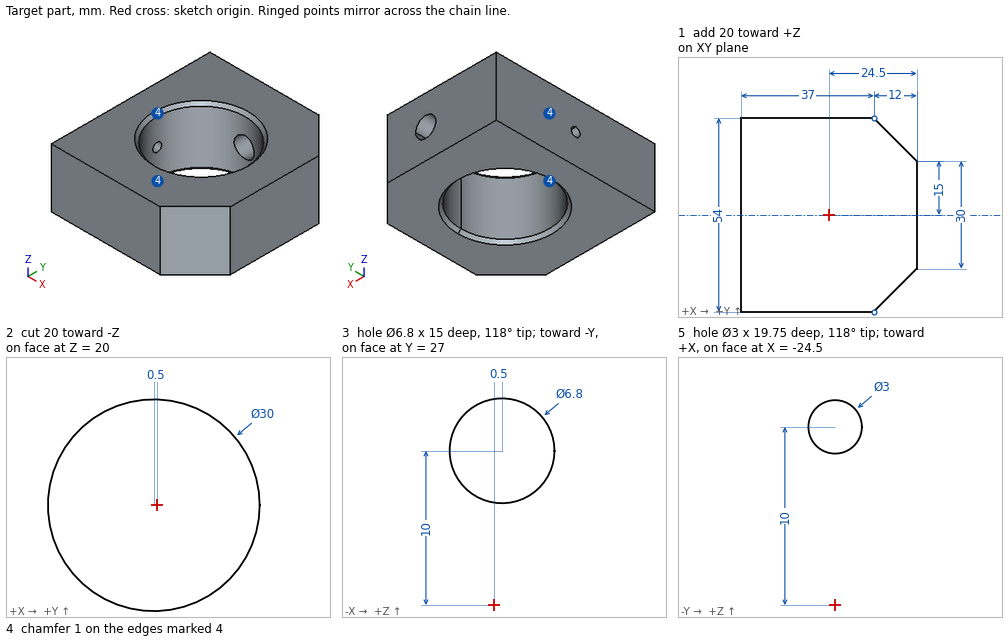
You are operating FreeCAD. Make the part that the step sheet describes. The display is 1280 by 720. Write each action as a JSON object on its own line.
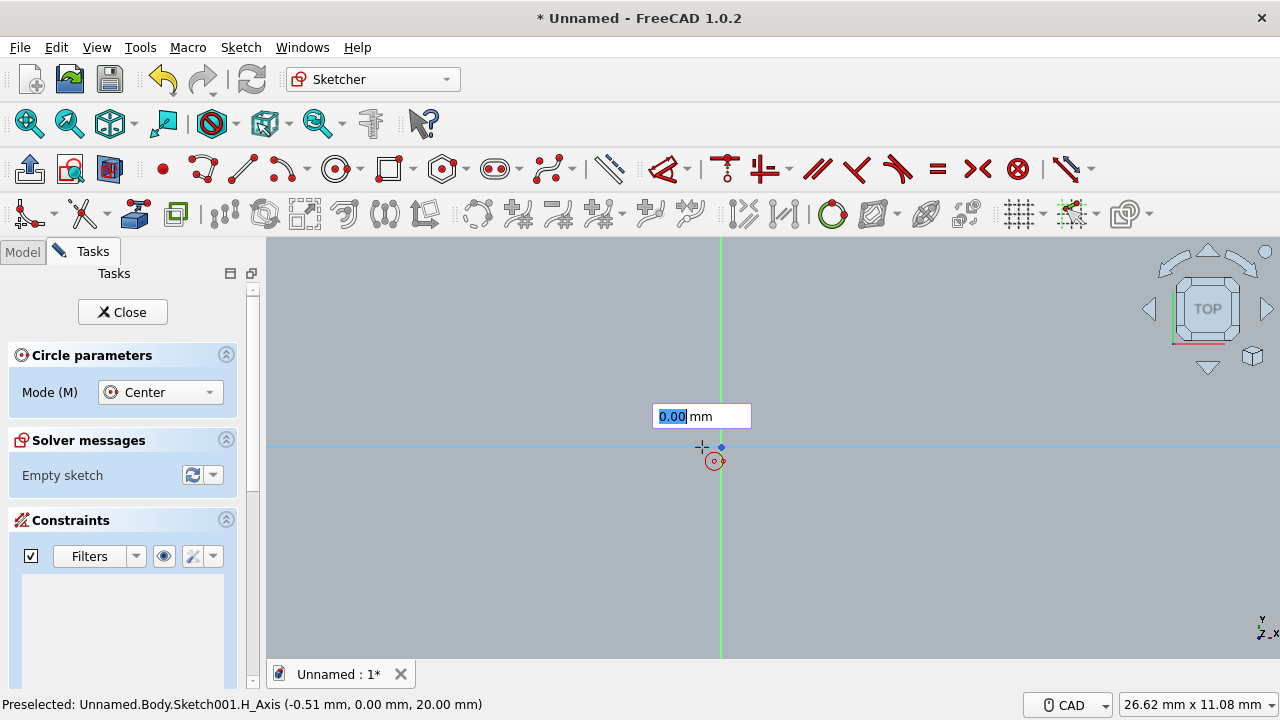
{"action": "scroll", "coordinate": [705, 448], "scroll_direction": "down", "scroll_amount": 7}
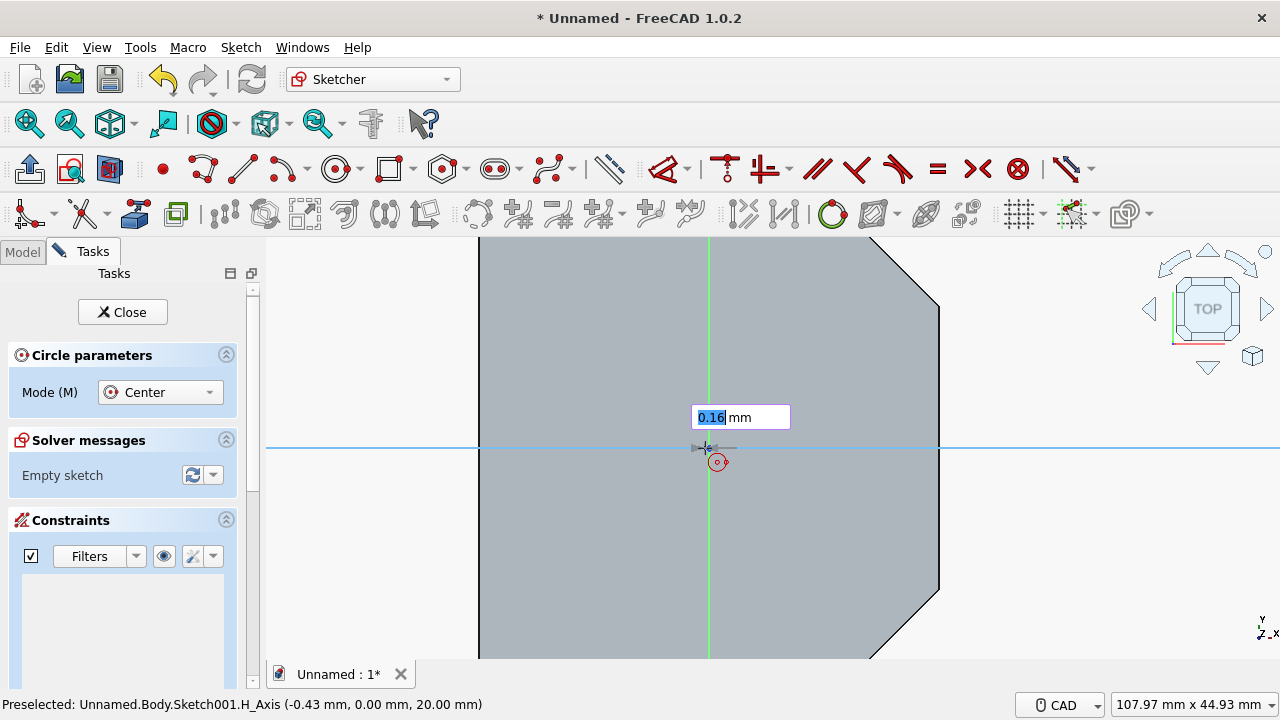
{"action": "left_click", "coordinate": [804, 349]}
{"action": "key", "text": "Escape"}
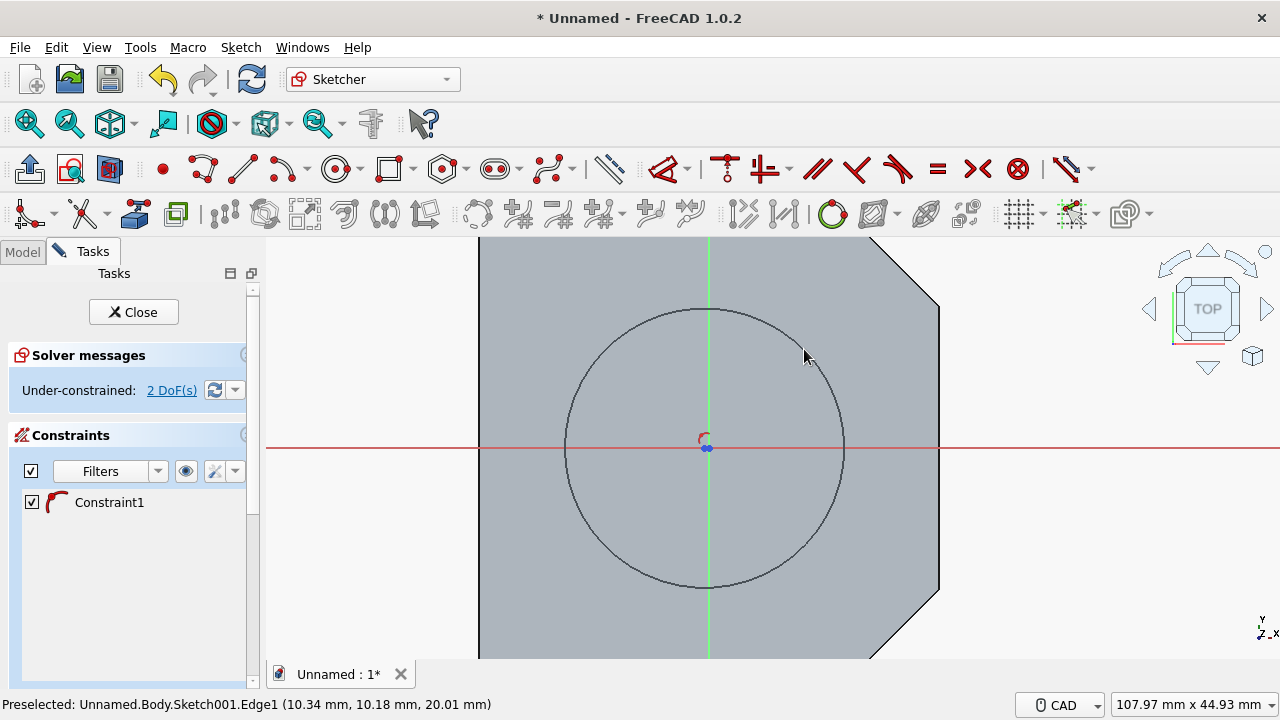
{"action": "key", "text": "d"}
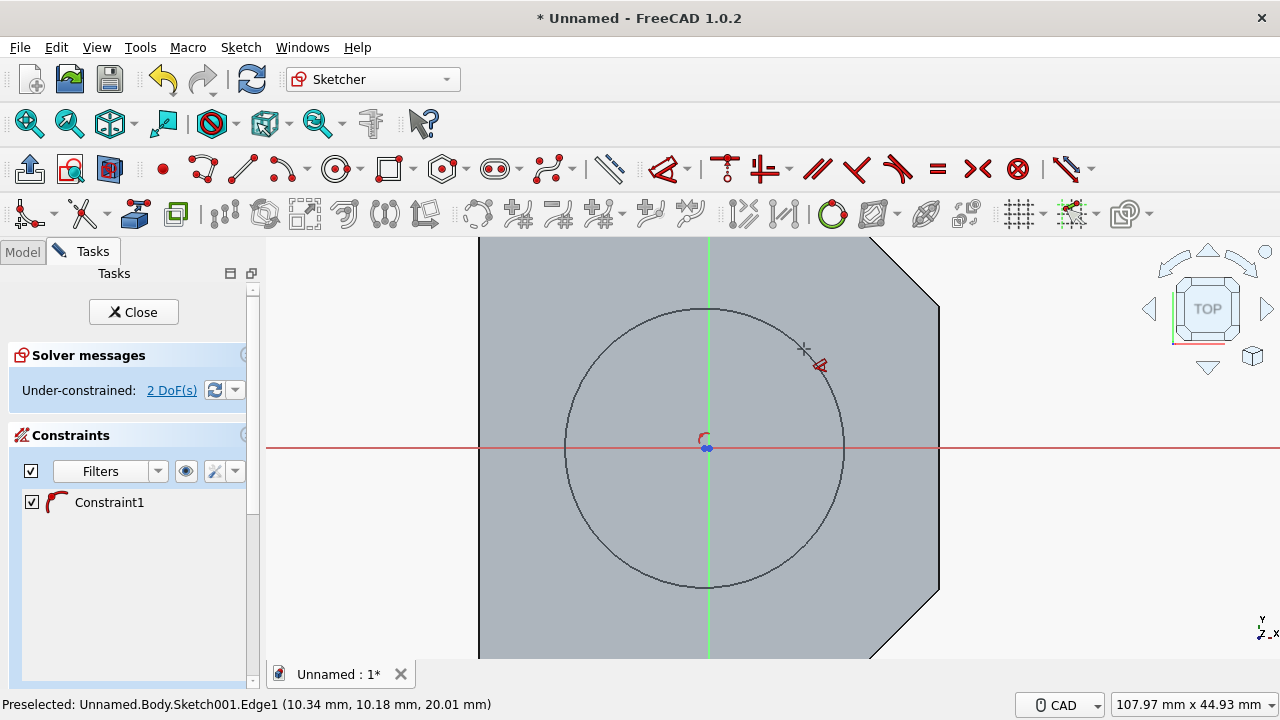
{"action": "left_click", "coordinate": [803, 349]}
{"action": "left_click", "coordinate": [826, 326]}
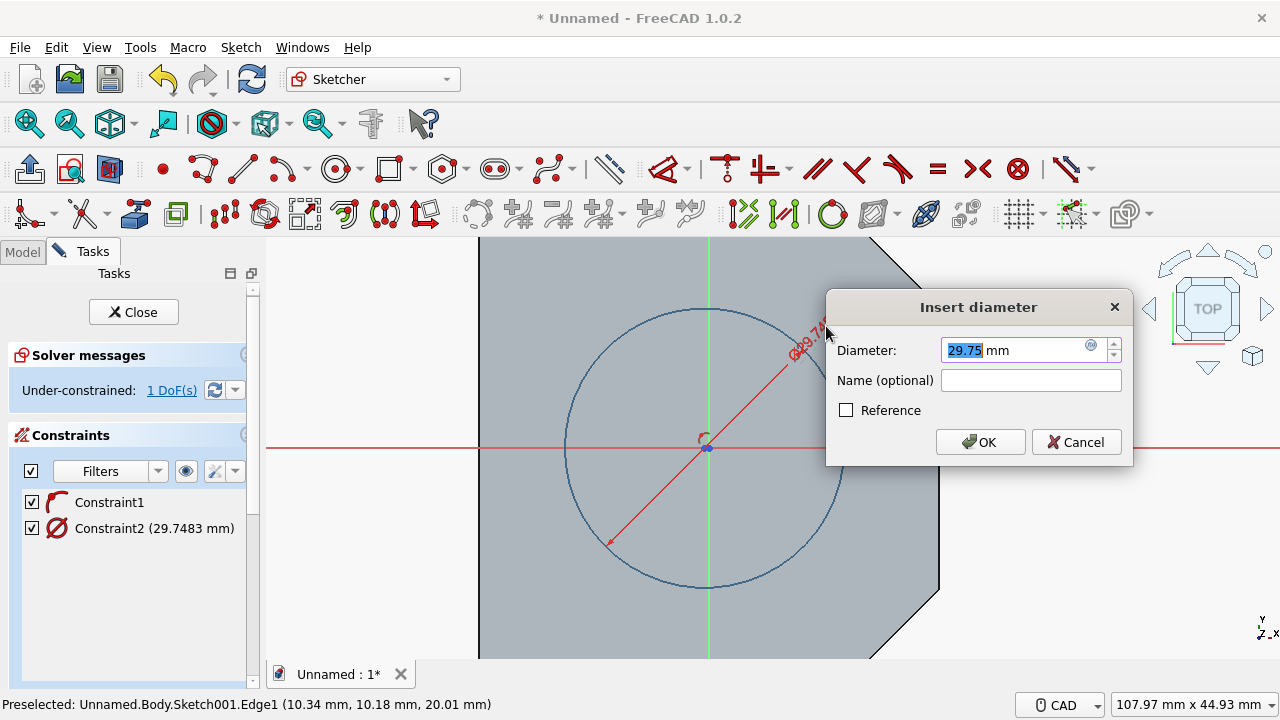
{"action": "type", "text": "30"}
{"action": "key", "text": "Return"}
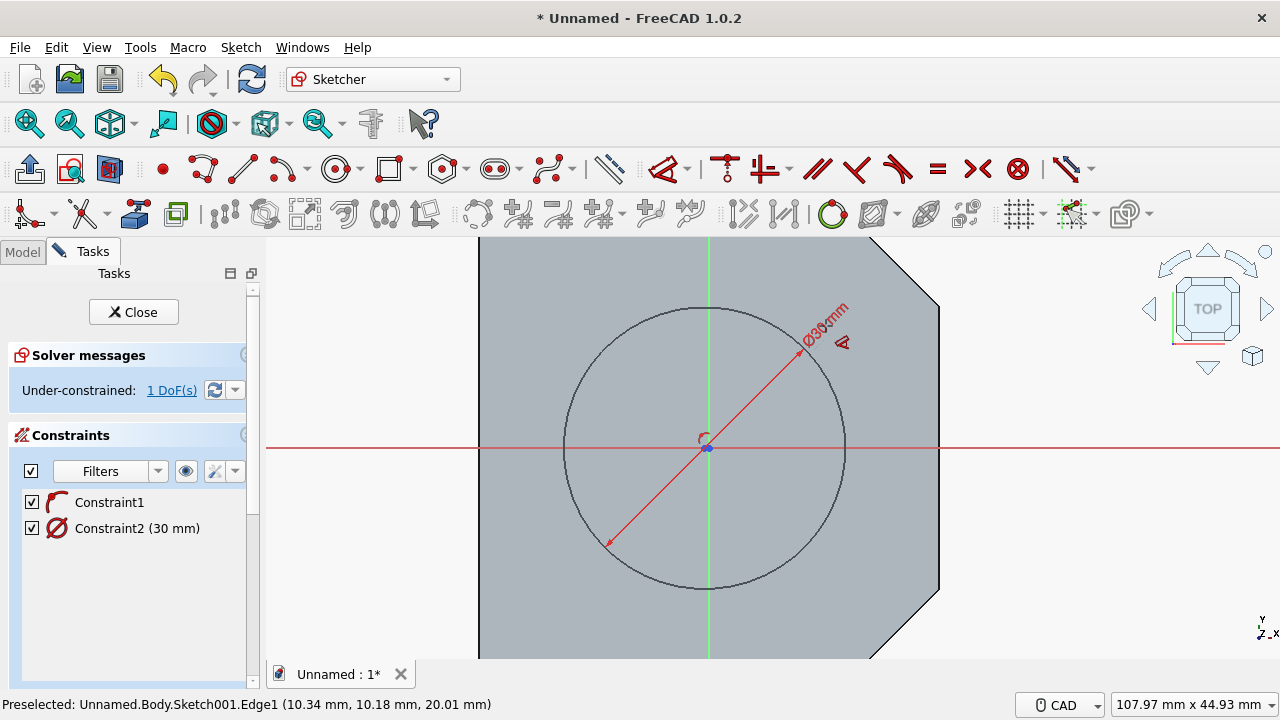
{"action": "scroll", "coordinate": [705, 448], "scroll_direction": "up", "scroll_amount": 11}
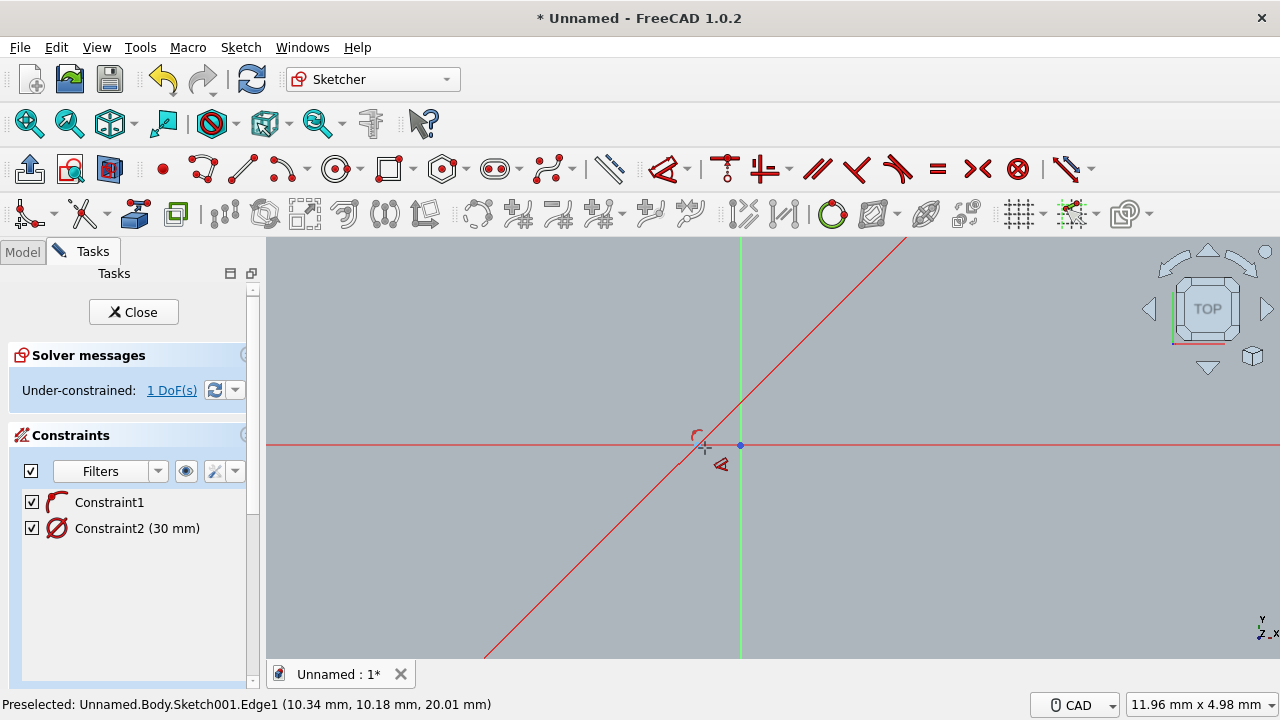
{"action": "left_click", "coordinate": [698, 445]}
{"action": "left_click", "coordinate": [719, 479]}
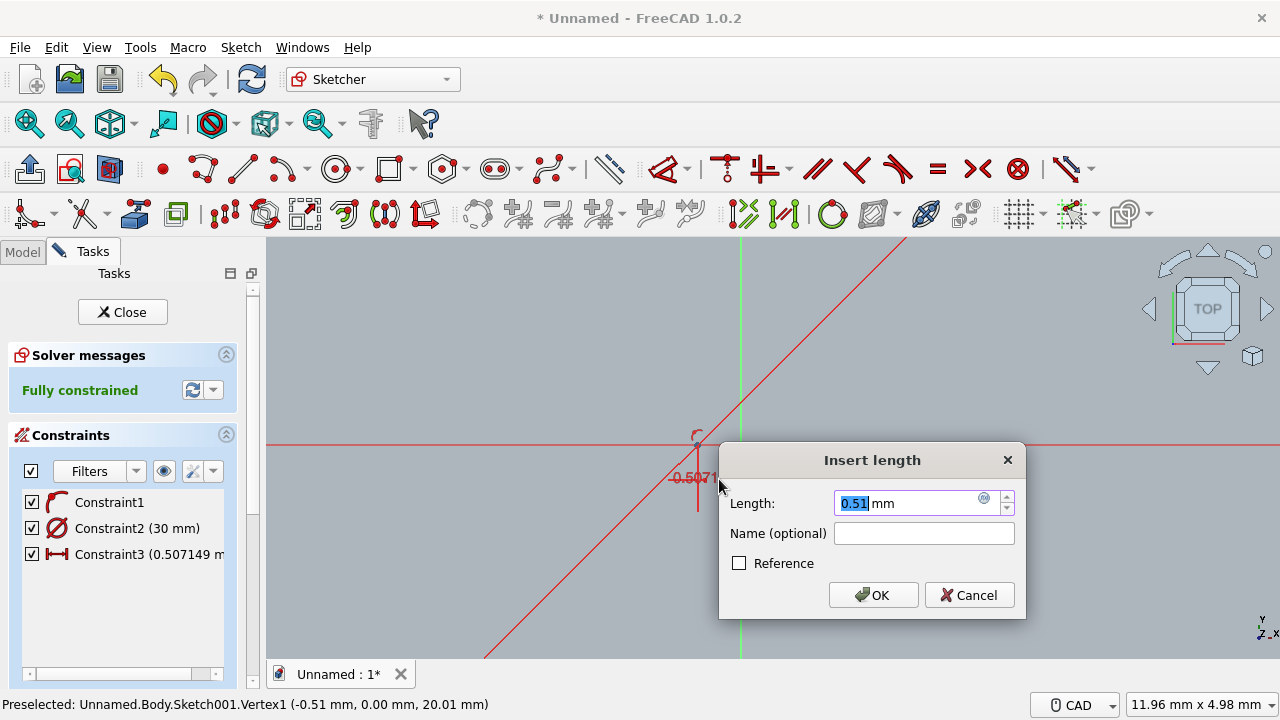
{"action": "type", "text": "0.5"}
{"action": "key", "text": "Return"}
{"action": "key", "text": "Escape"}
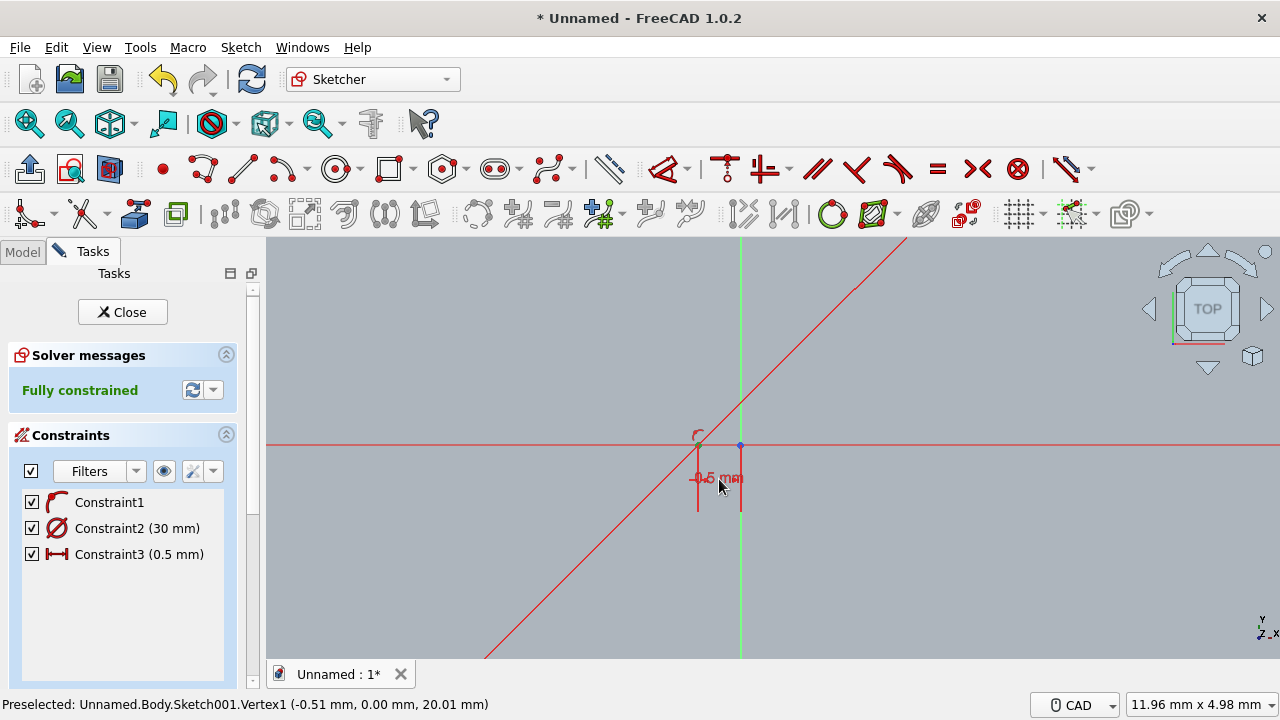
{"action": "left_click", "coordinate": [123, 312]}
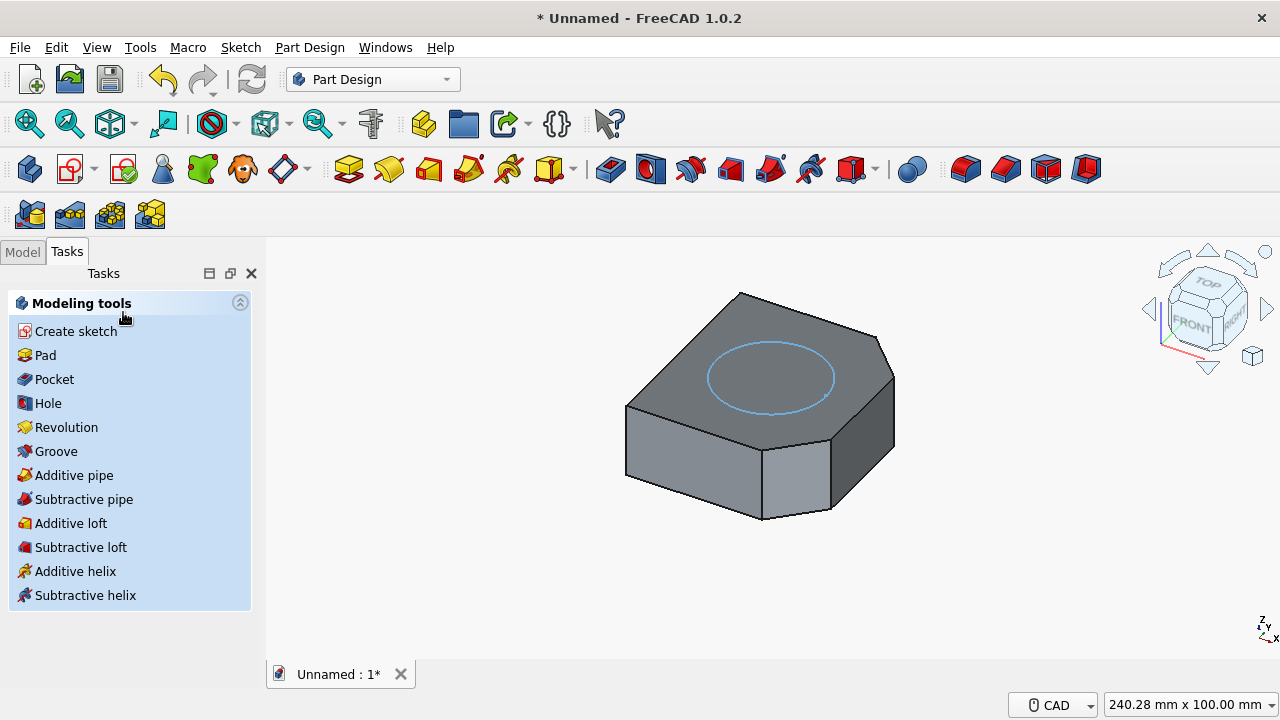
{"action": "left_click", "coordinate": [612, 170]}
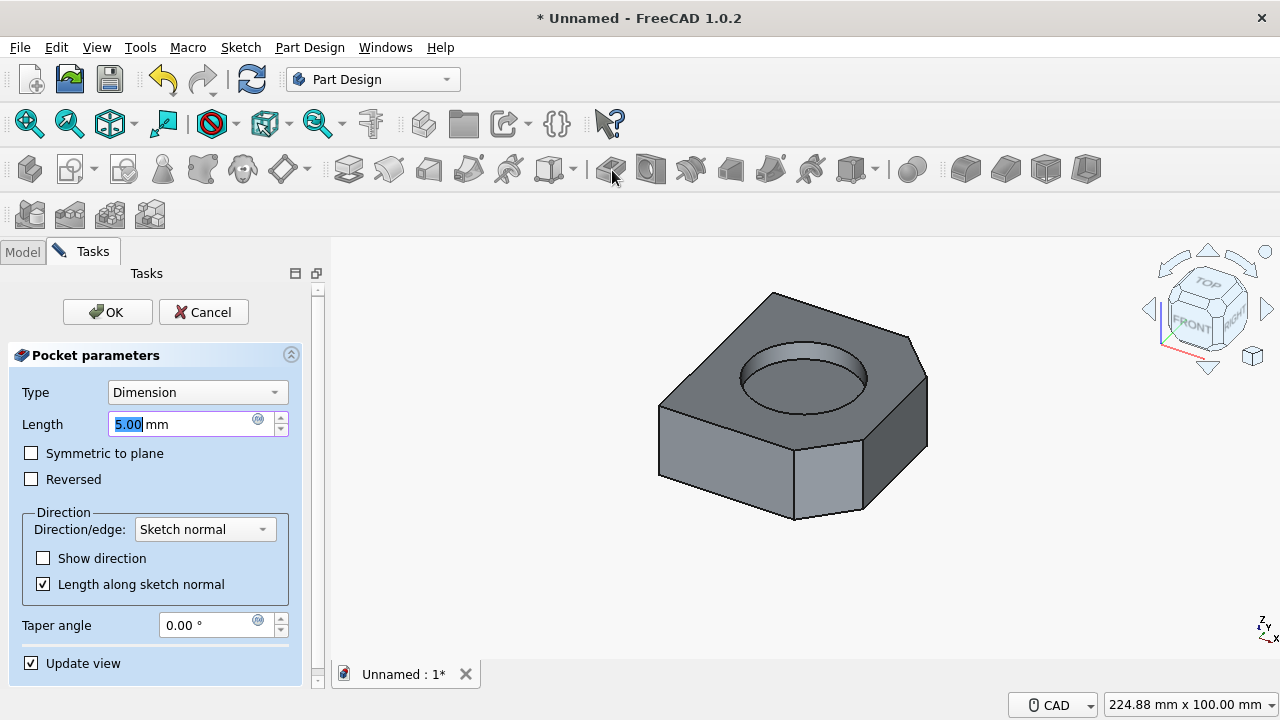
{"action": "type", "text": "20"}
{"action": "key", "text": "Tab"}